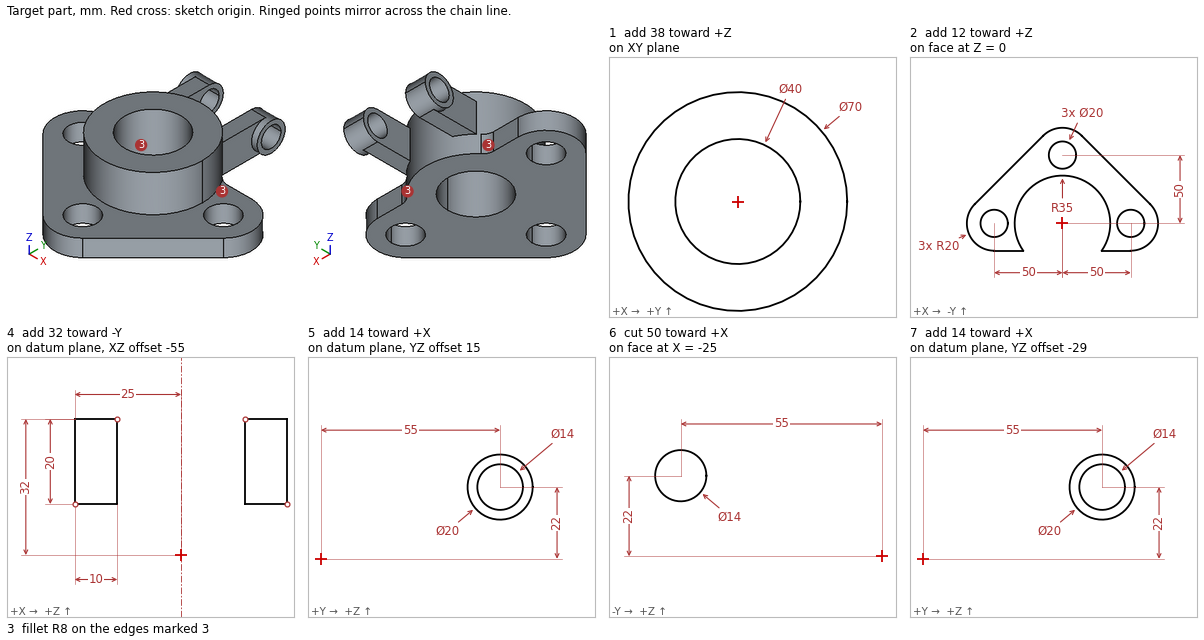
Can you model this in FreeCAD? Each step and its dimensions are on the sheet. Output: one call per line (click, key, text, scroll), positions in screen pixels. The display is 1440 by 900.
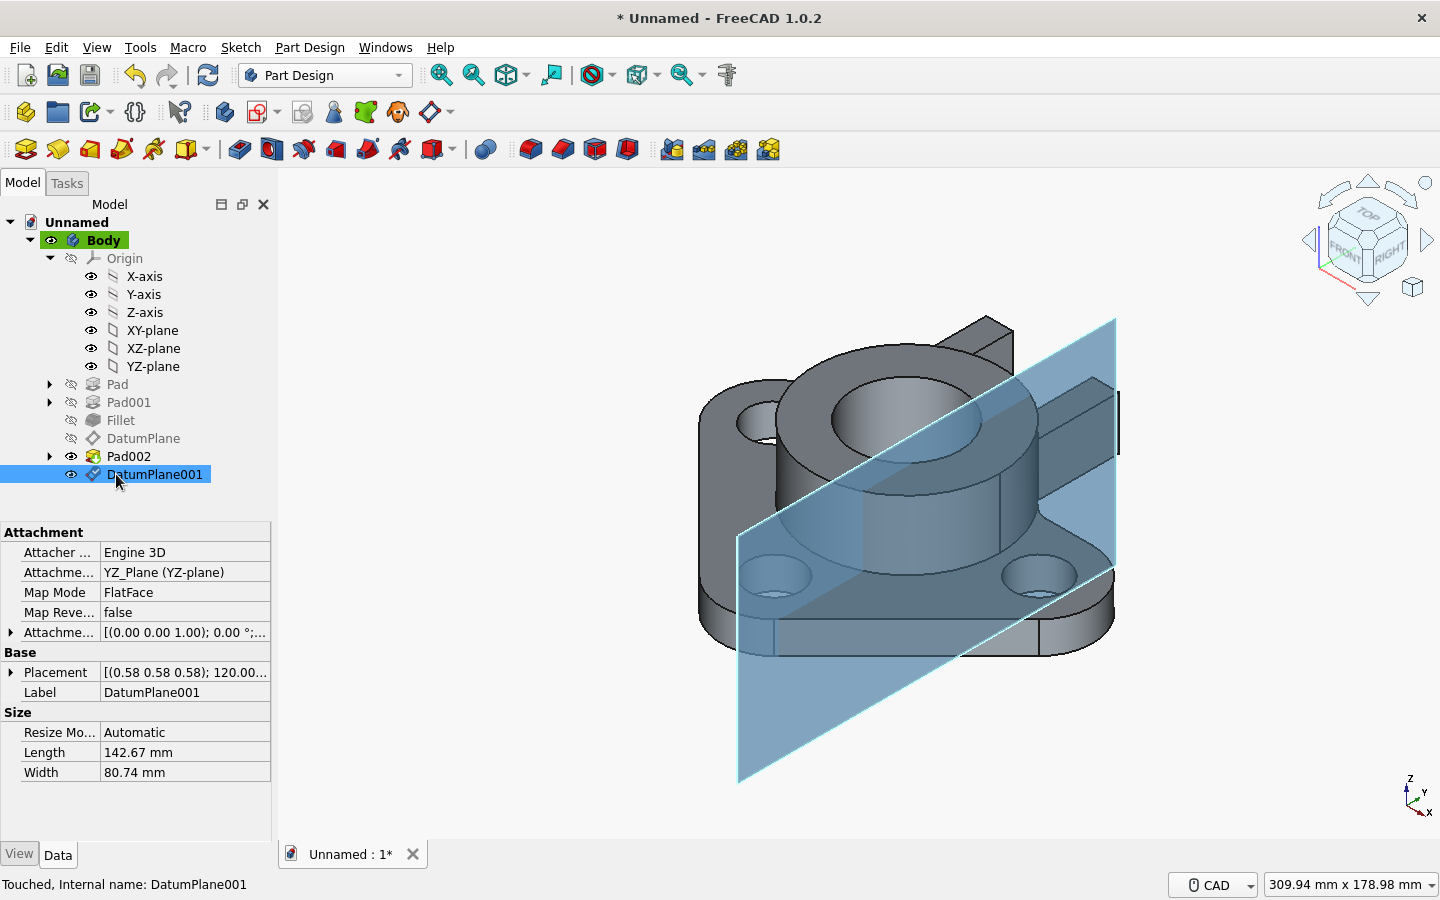
click(258, 112)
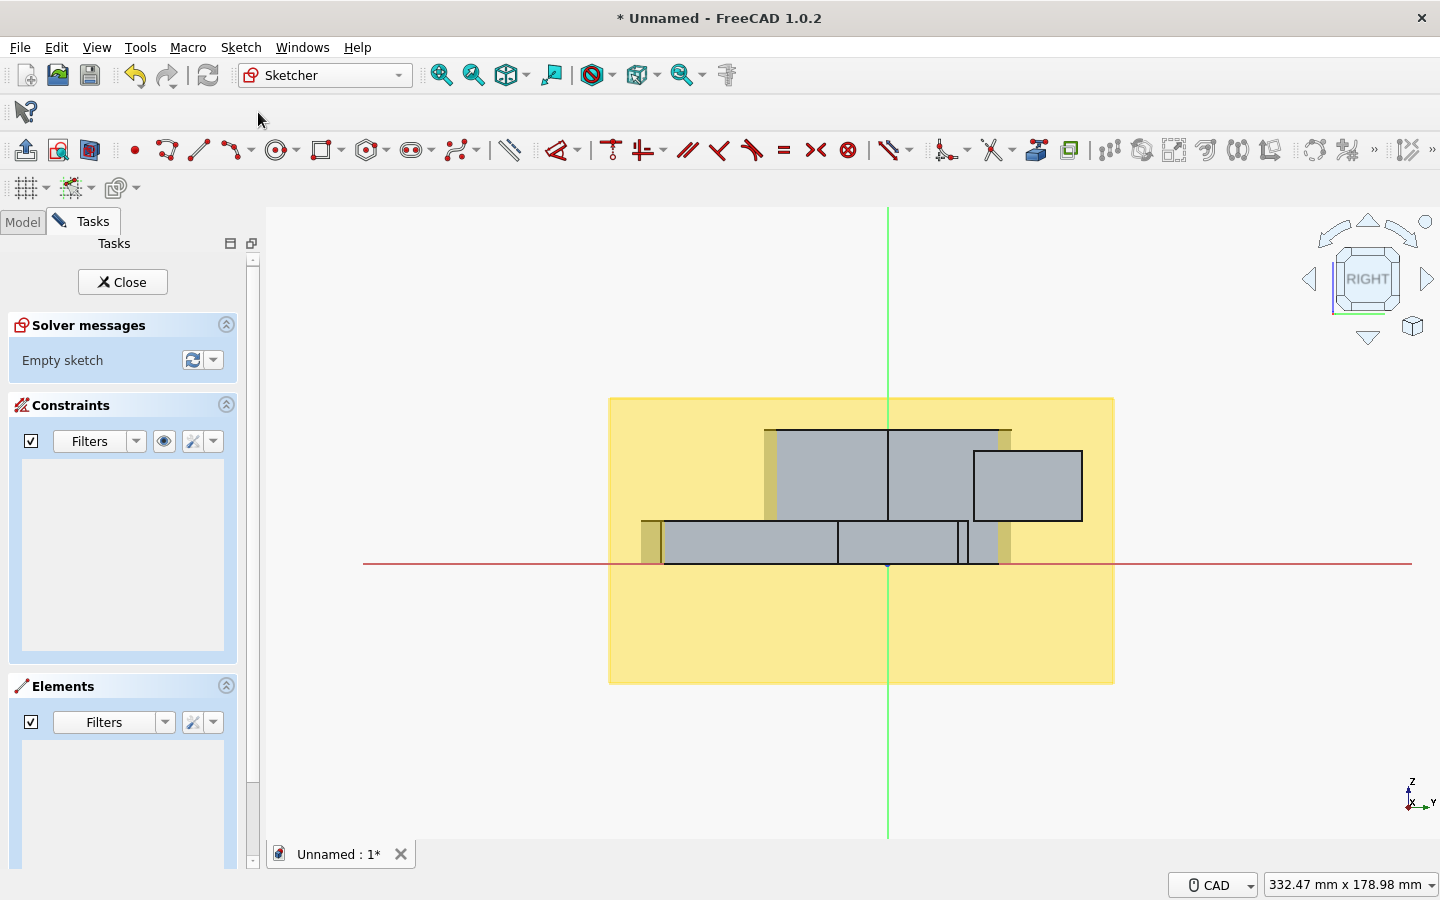
click(90, 150)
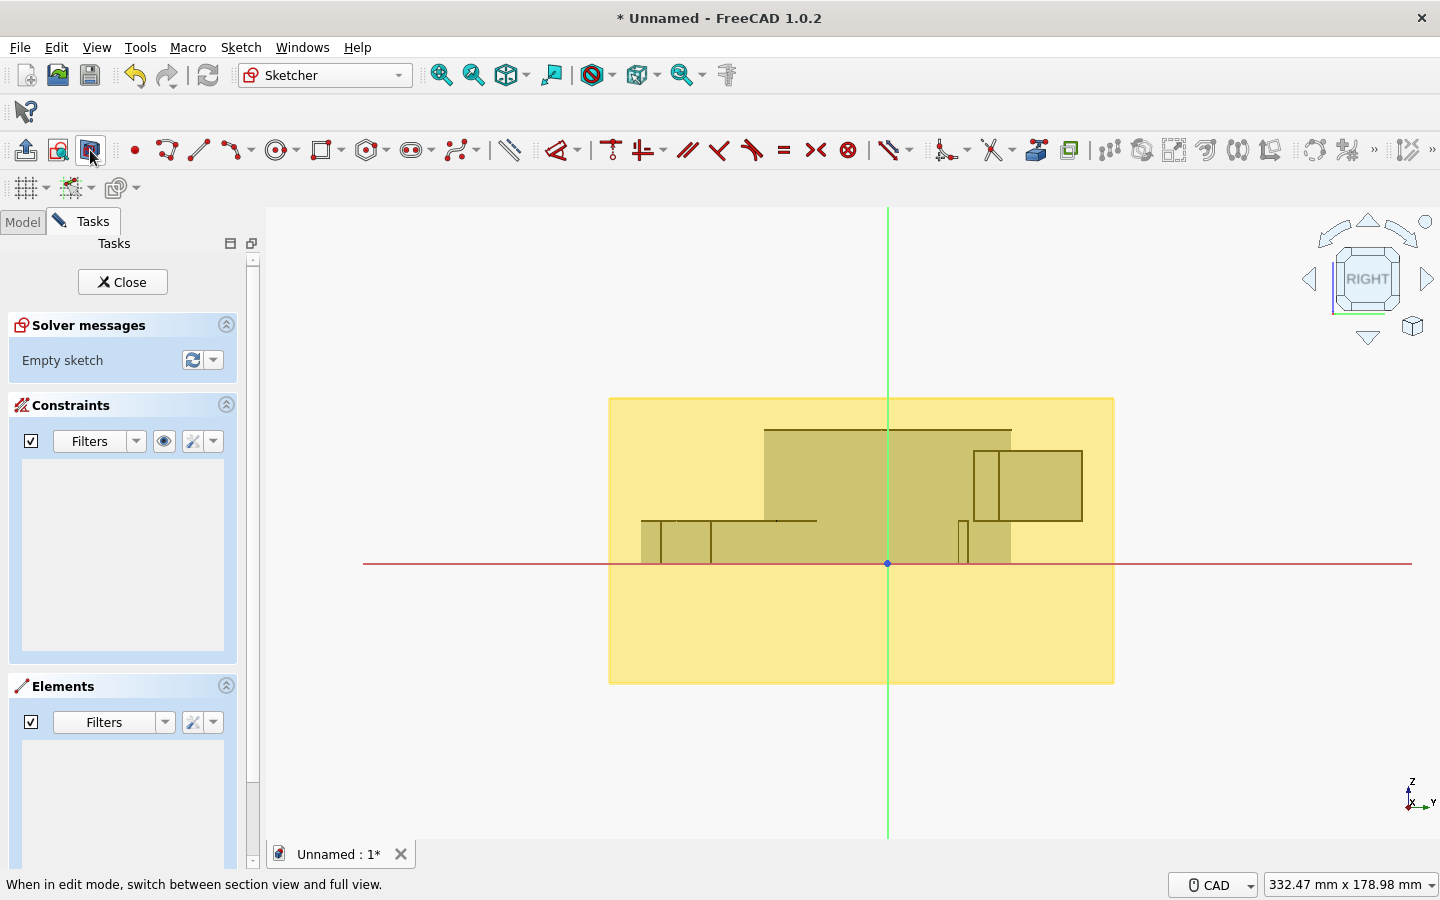
scroll(1141, 479, up, 9)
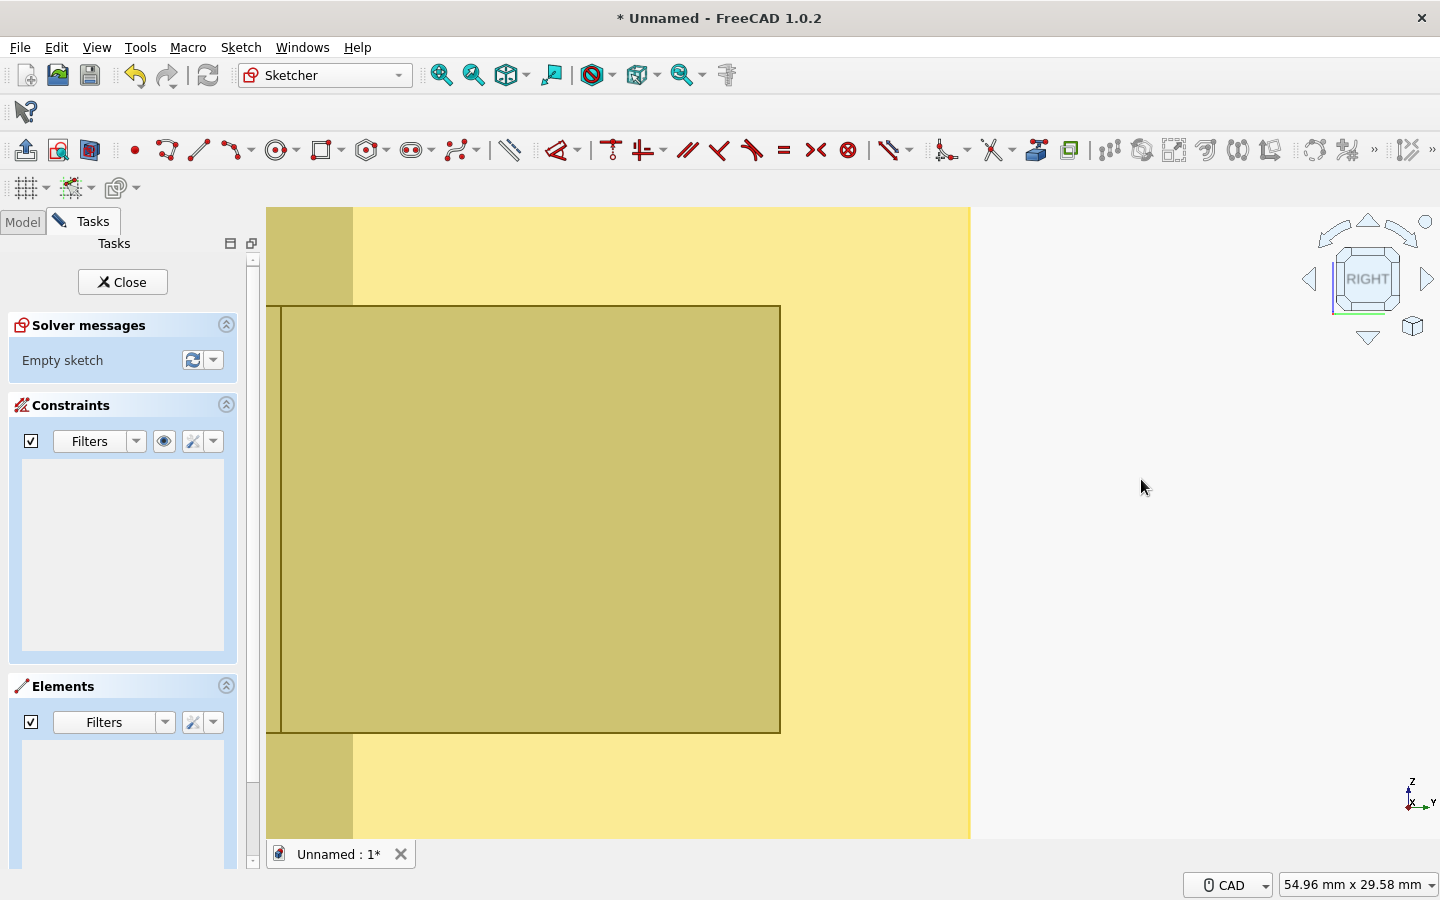
click(276, 150)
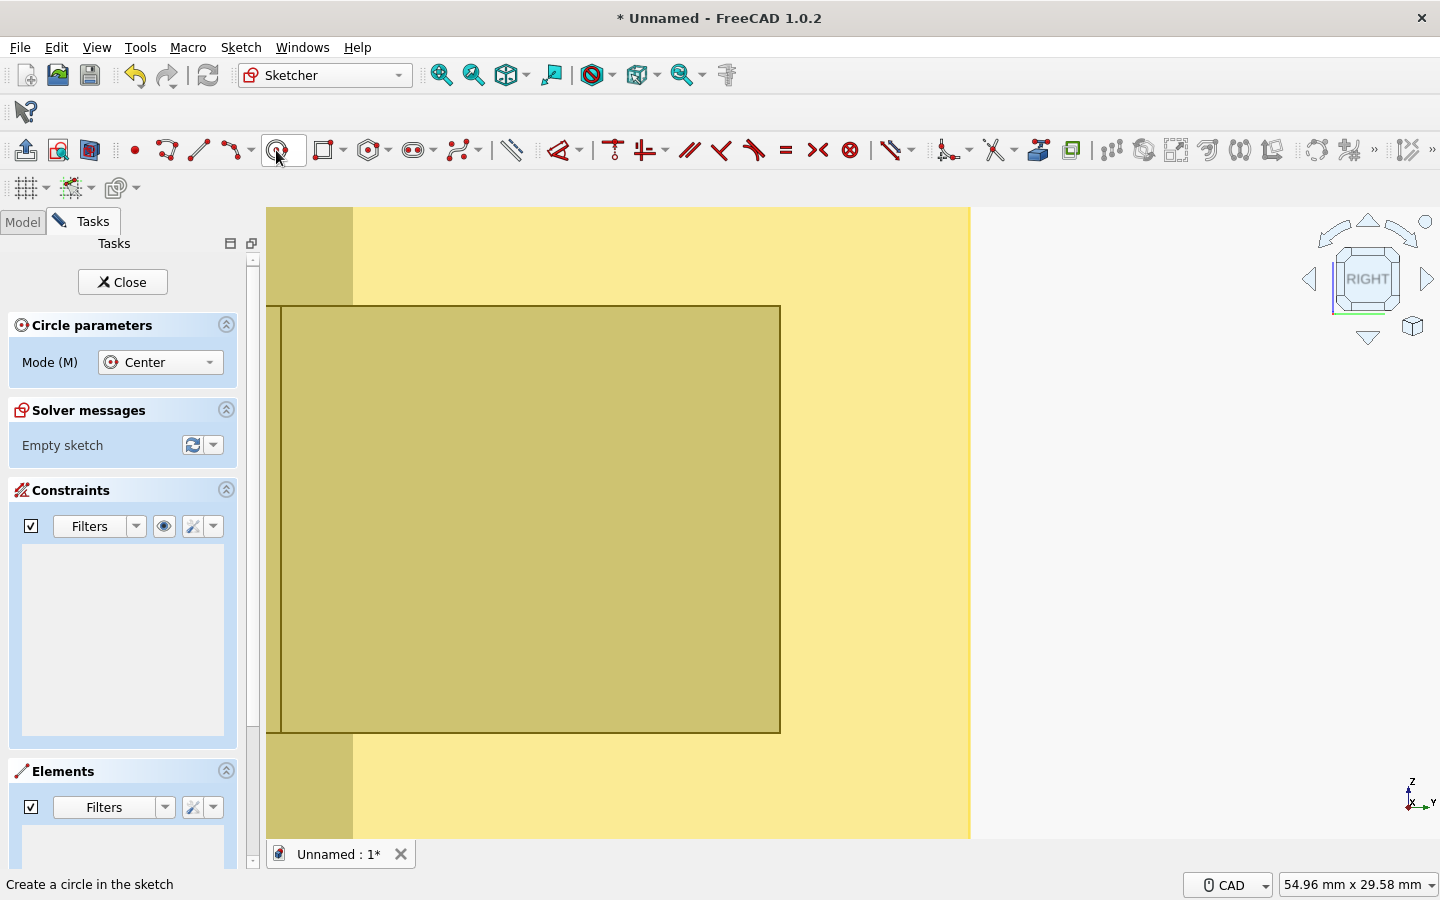
click(780, 519)
click(931, 368)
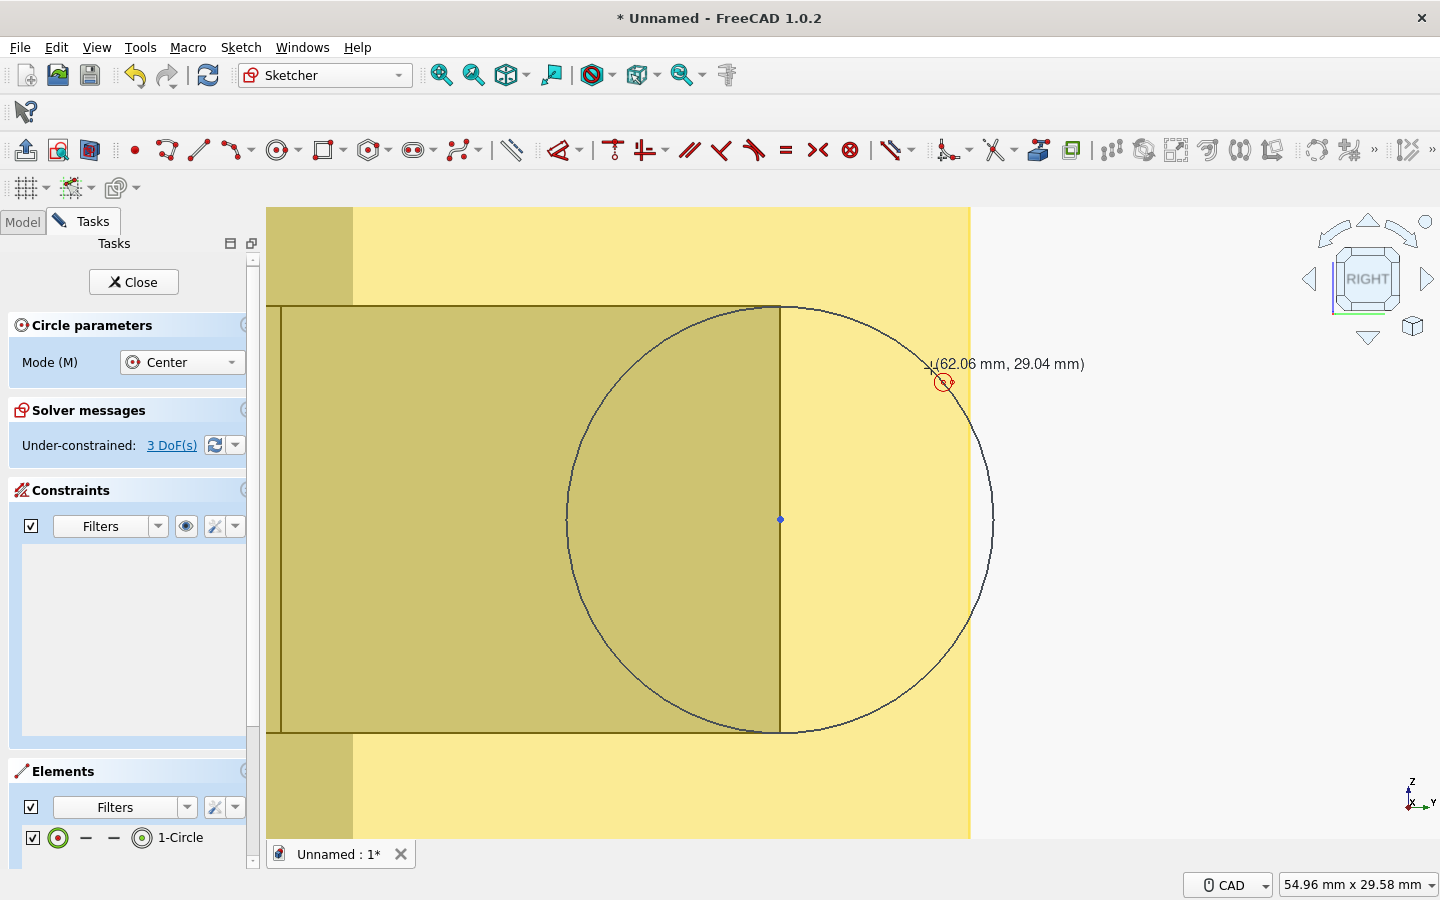
click(780, 520)
click(886, 414)
key(Escape)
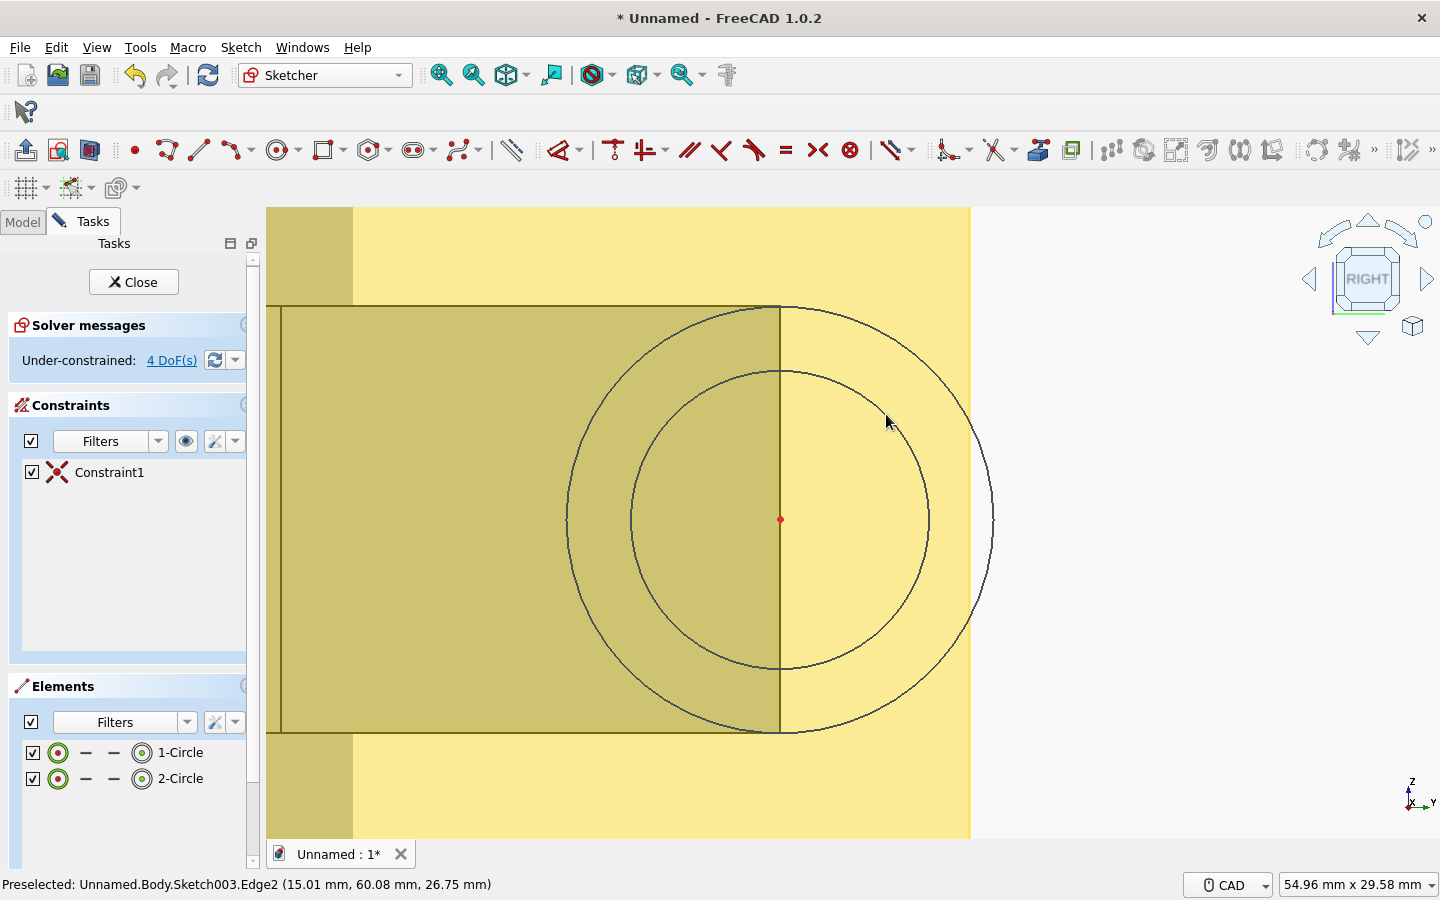
key(d)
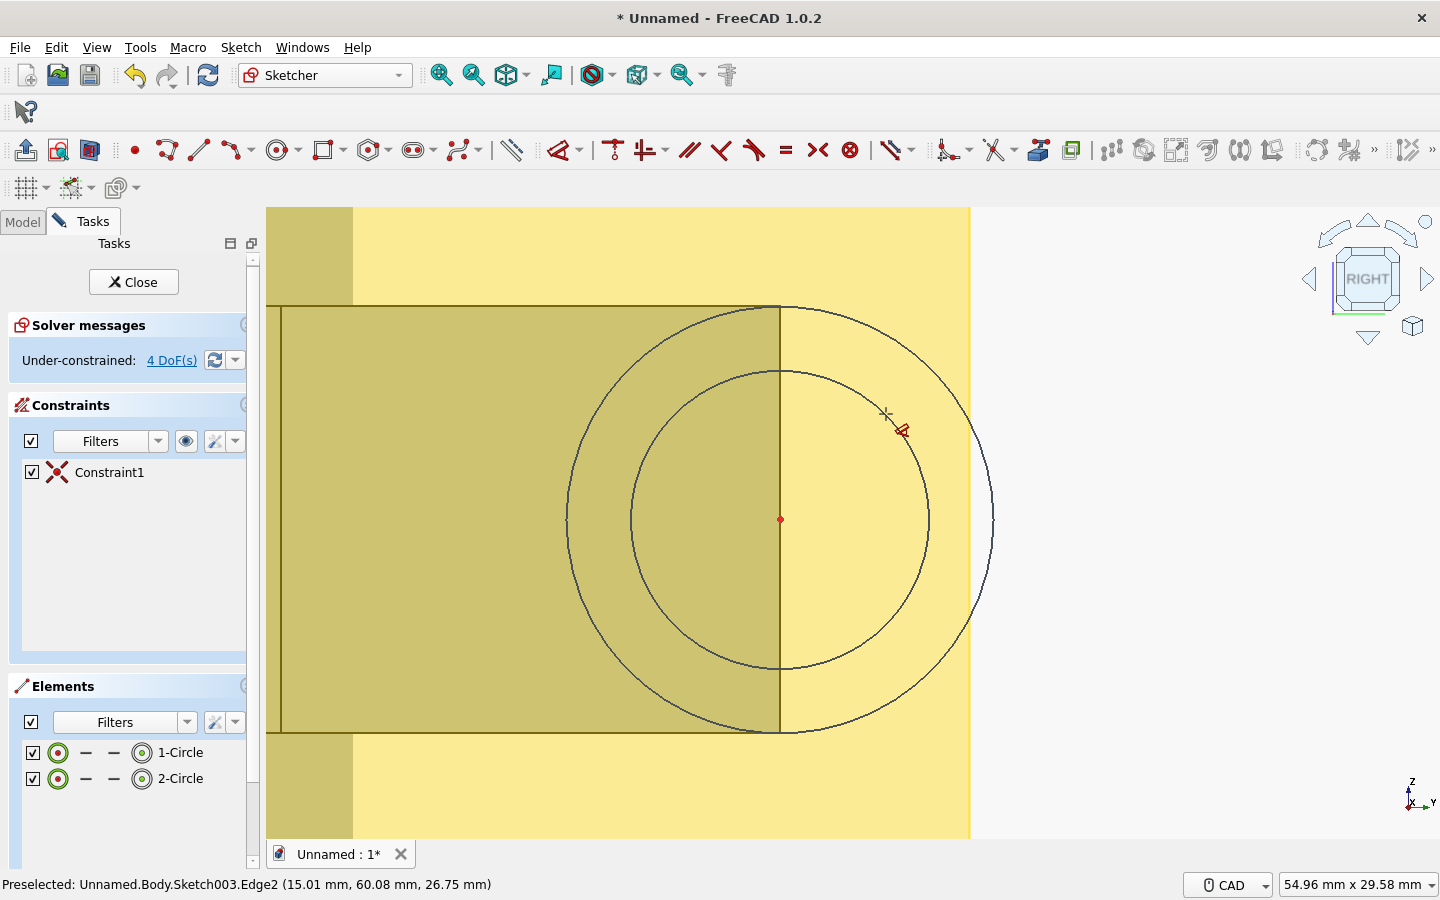
click(931, 369)
click(954, 346)